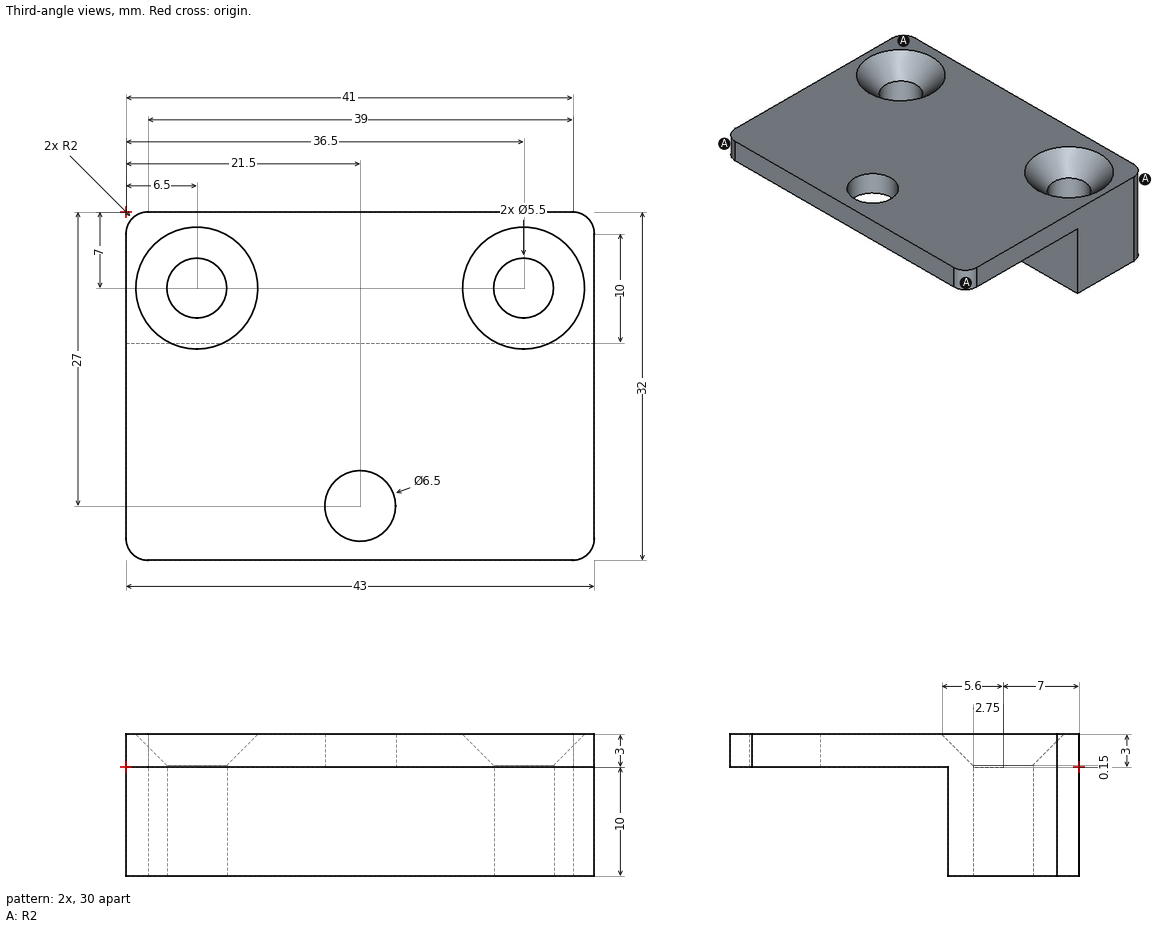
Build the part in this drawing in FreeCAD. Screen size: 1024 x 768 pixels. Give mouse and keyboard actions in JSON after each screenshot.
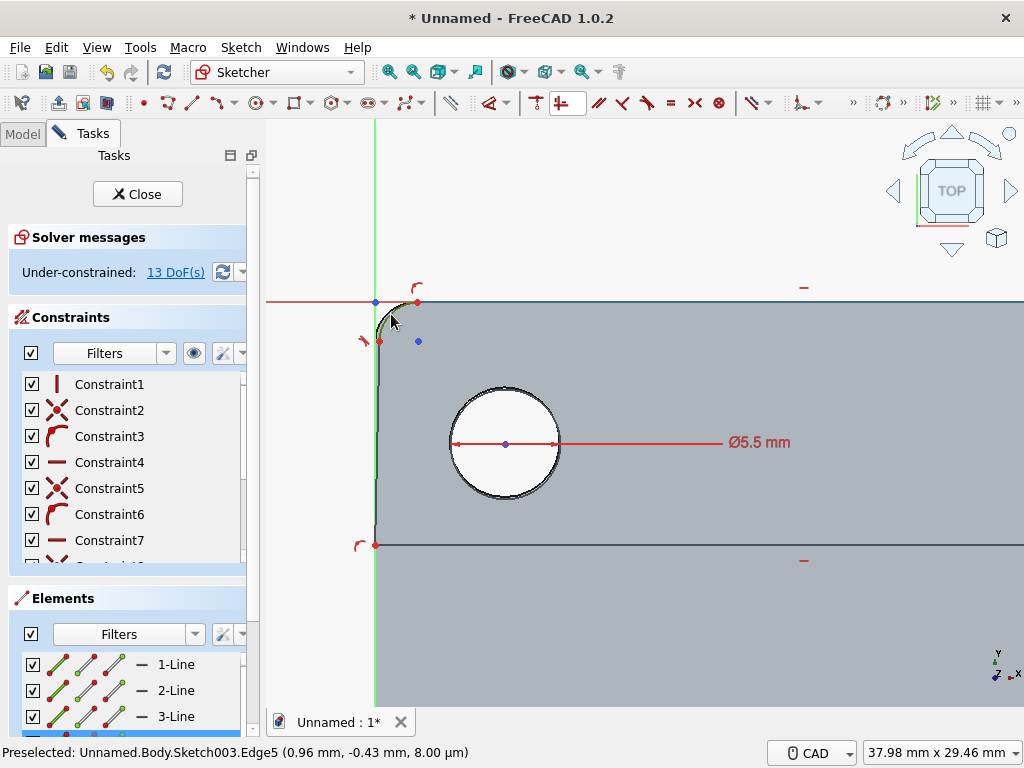
{"action": "left_click", "coordinate": [648, 104]}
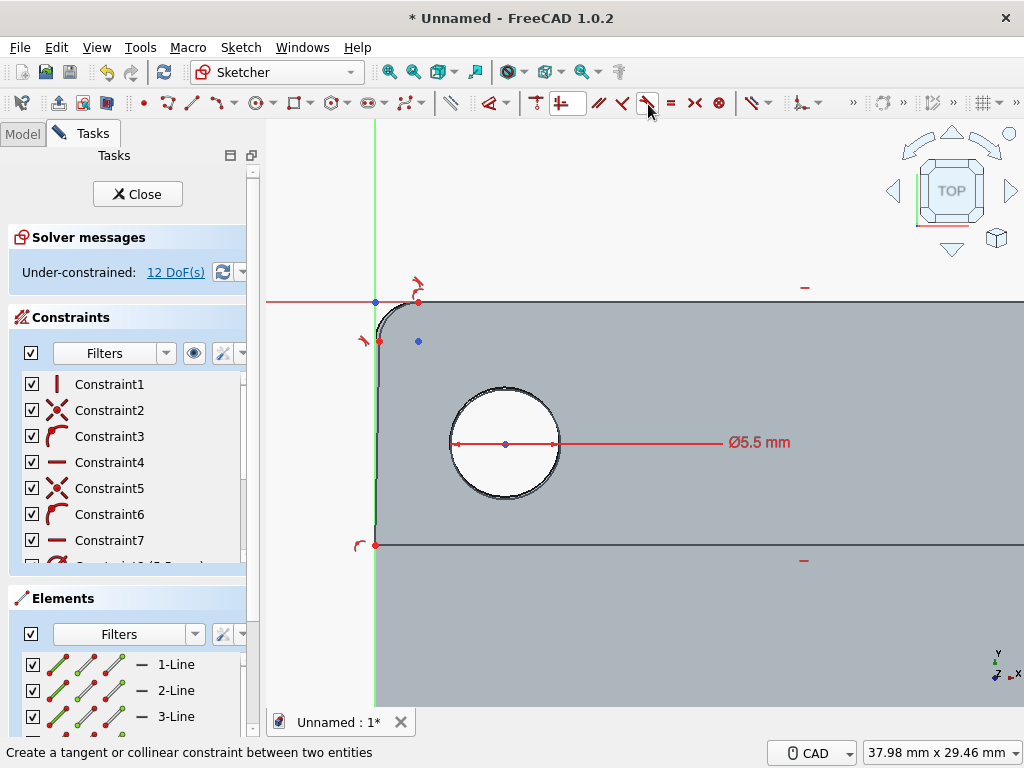
{"action": "left_click", "coordinate": [651, 302]}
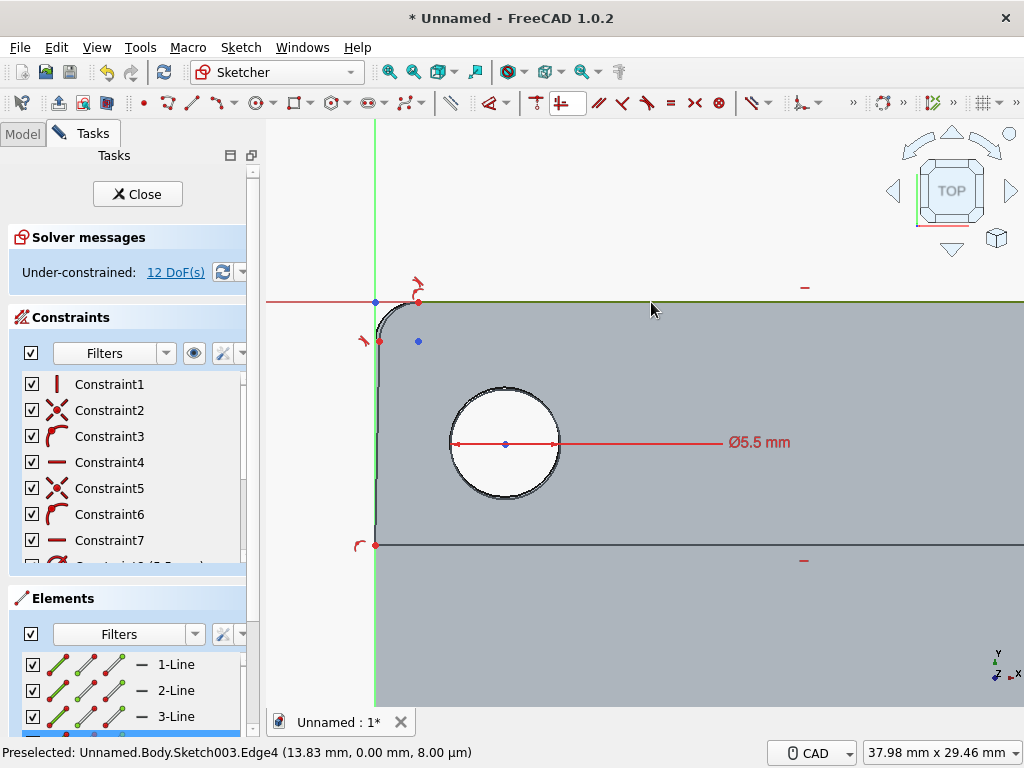
{"action": "scroll", "coordinate": [391, 405], "scroll_direction": "down", "scroll_amount": 4}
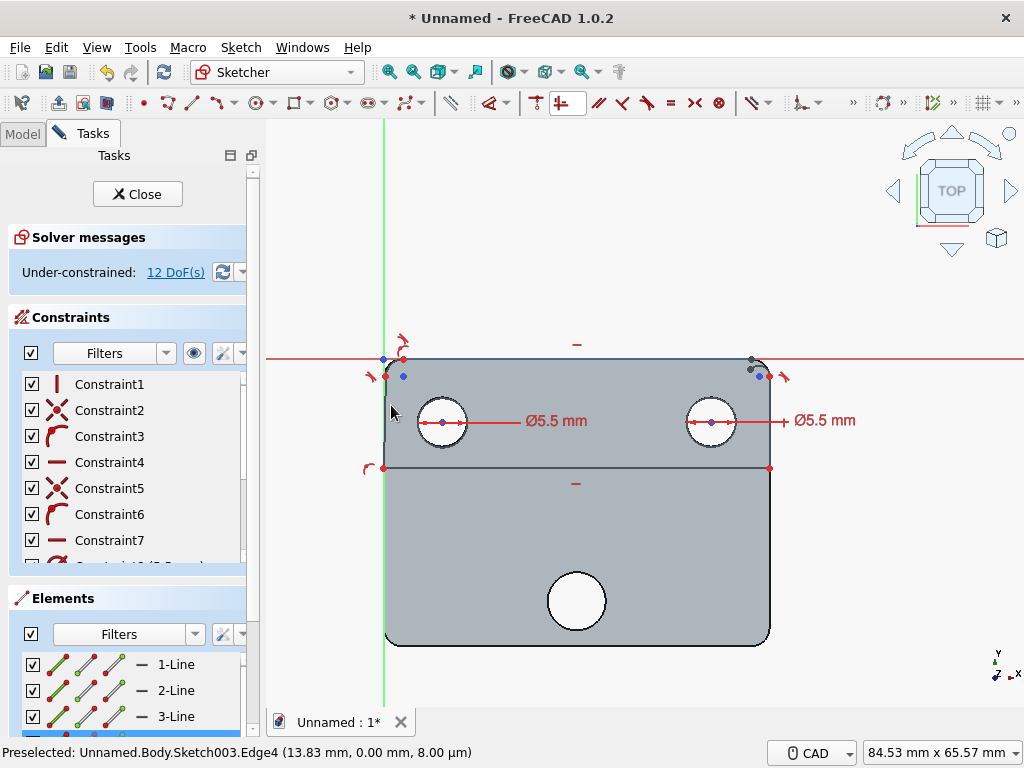
{"action": "scroll", "coordinate": [767, 369], "scroll_direction": "up", "scroll_amount": 3}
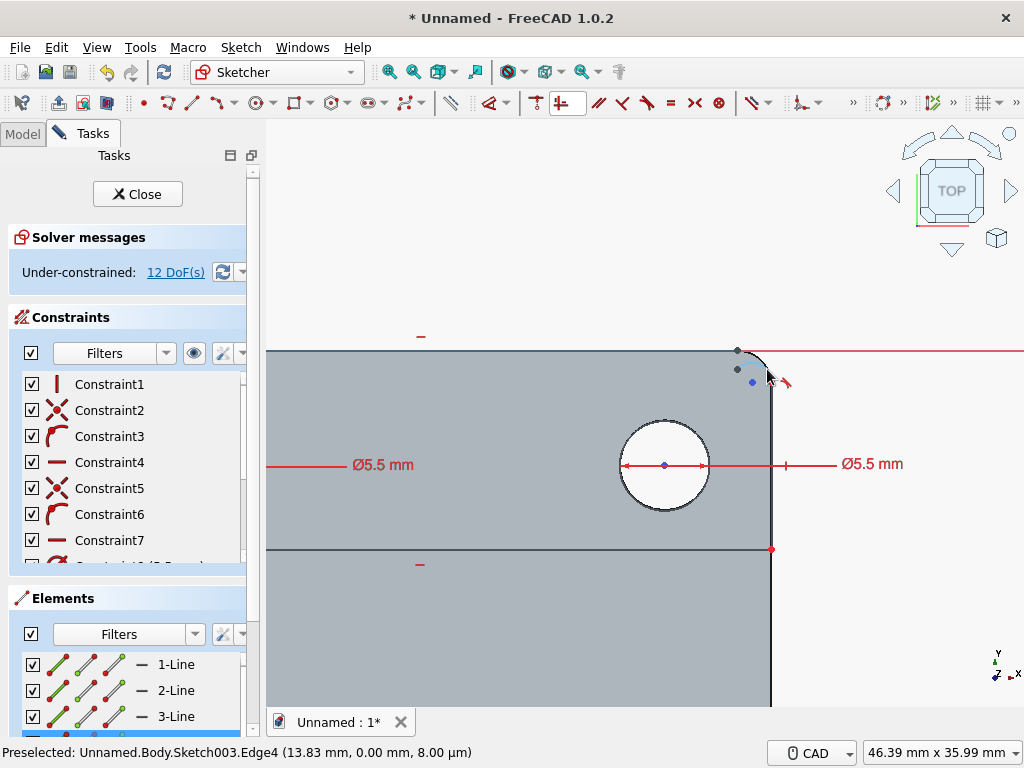
{"action": "left_click", "coordinate": [767, 369]}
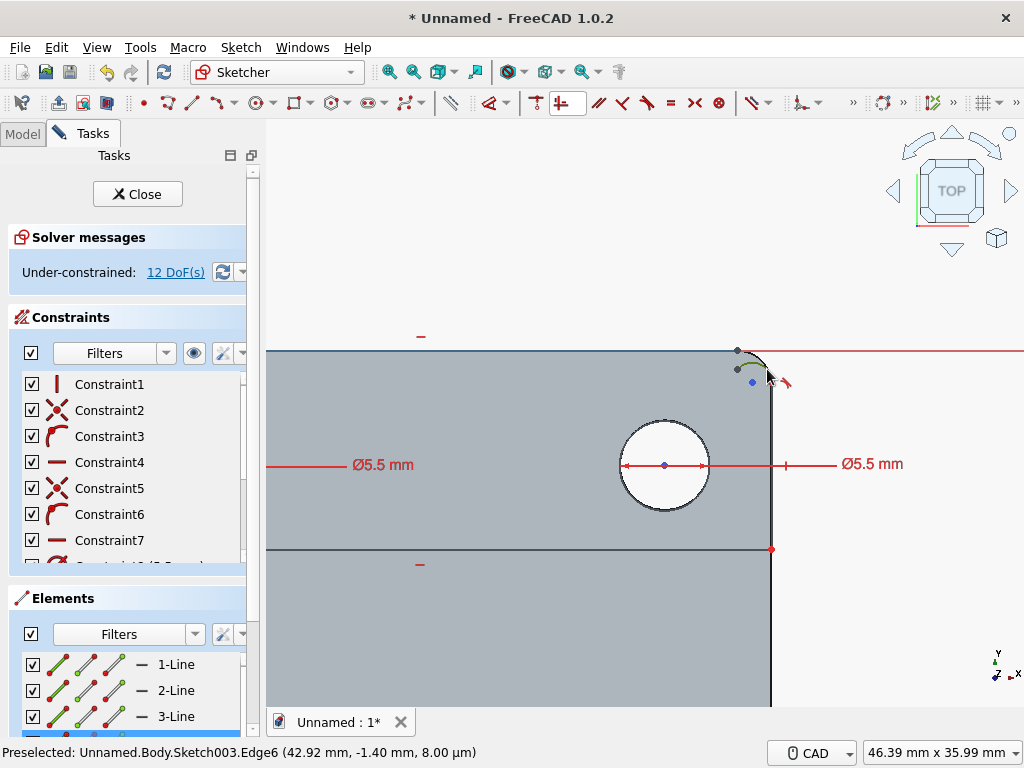
{"action": "left_click", "coordinate": [648, 104]}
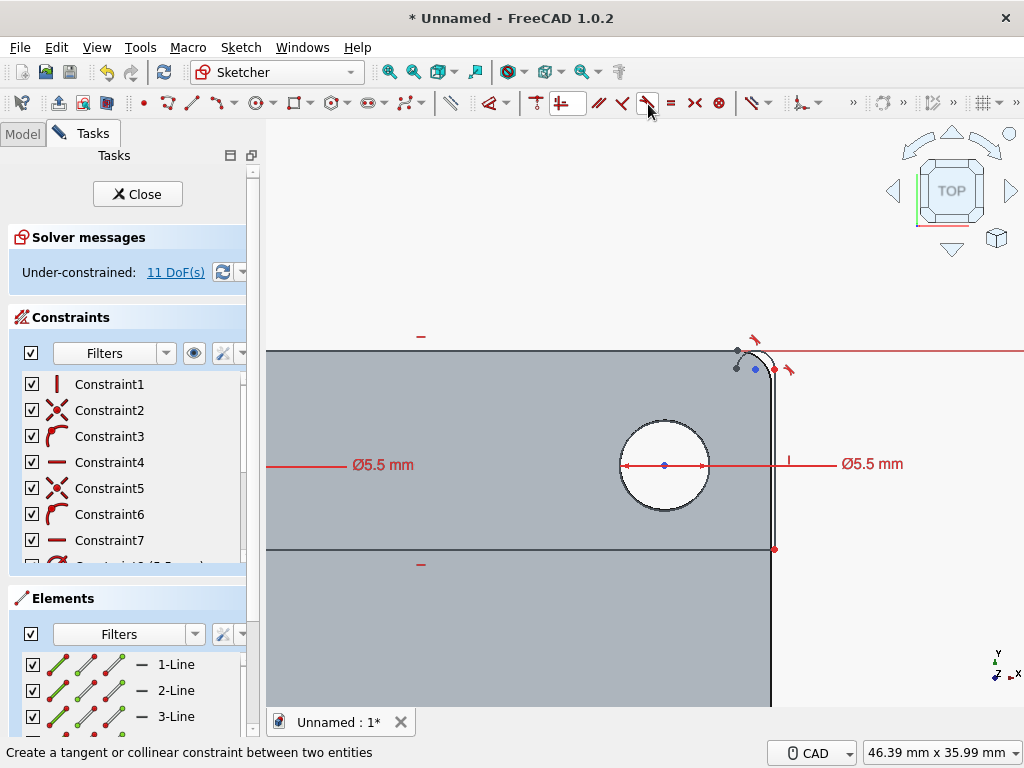
{"action": "scroll", "coordinate": [767, 369], "scroll_direction": "down", "scroll_amount": 3}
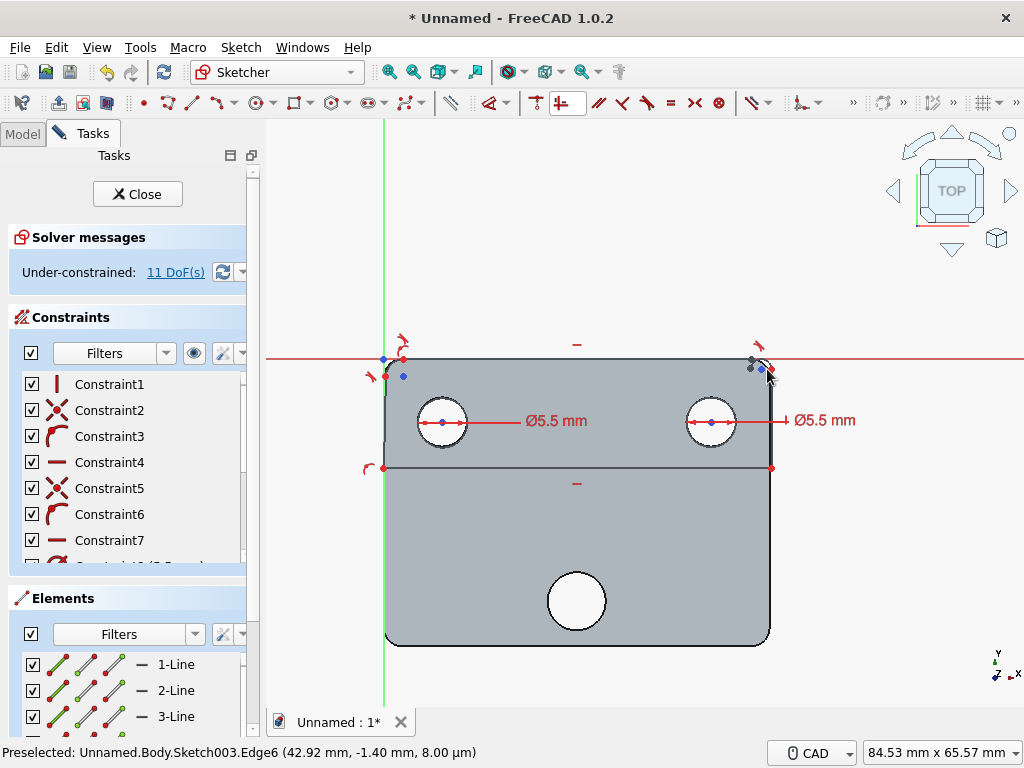
{"action": "left_click", "coordinate": [385, 441]}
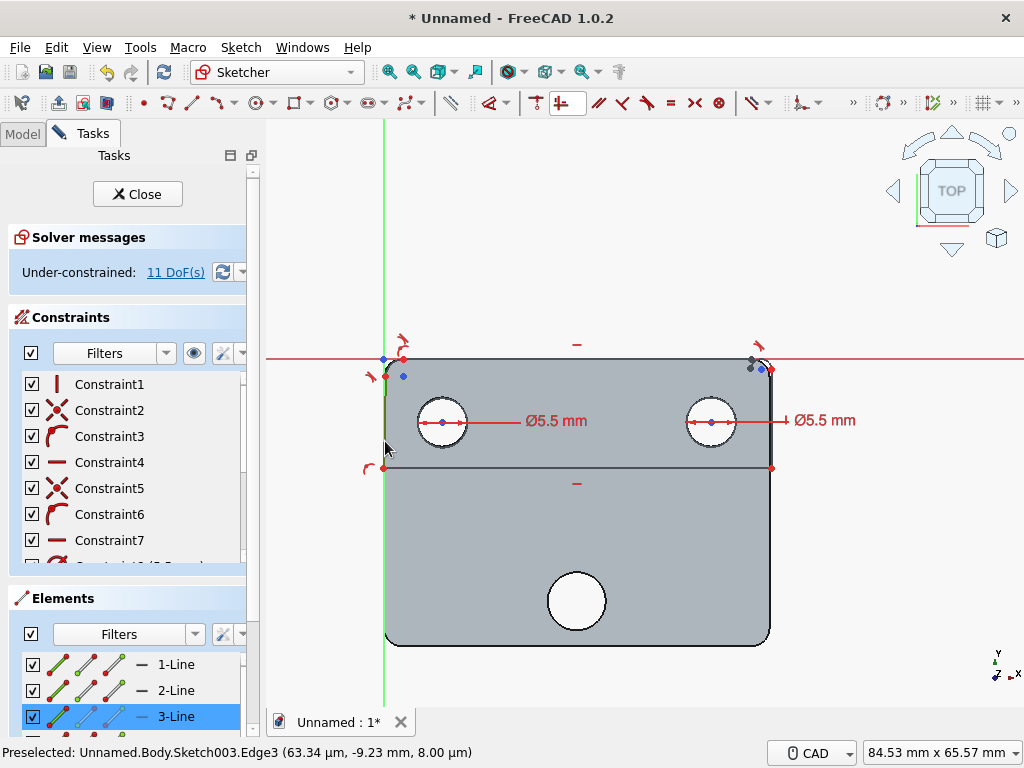
{"action": "left_click", "coordinate": [580, 104]}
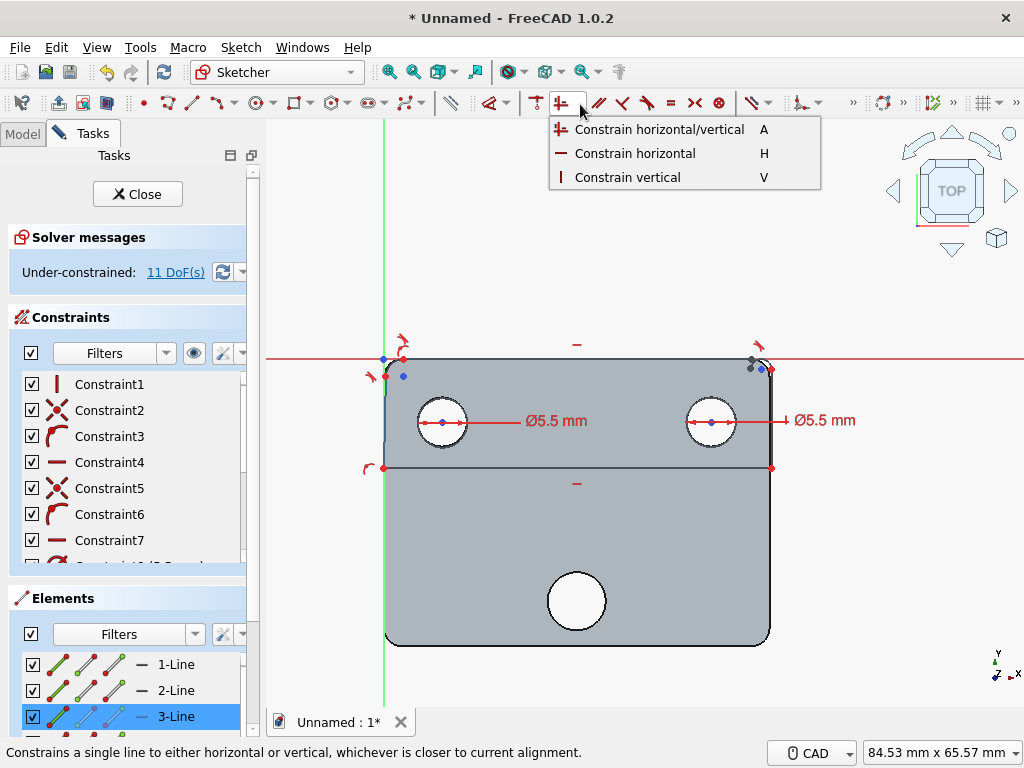
{"action": "left_click", "coordinate": [685, 177]}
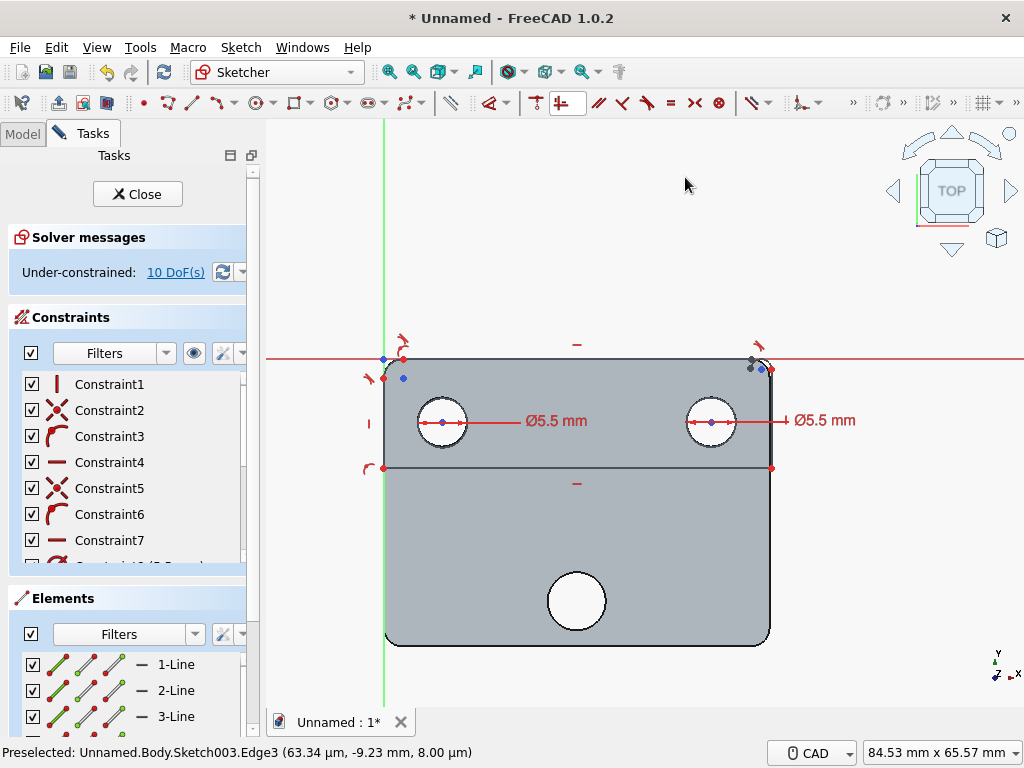
{"action": "scroll", "coordinate": [395, 361], "scroll_direction": "up", "scroll_amount": 3}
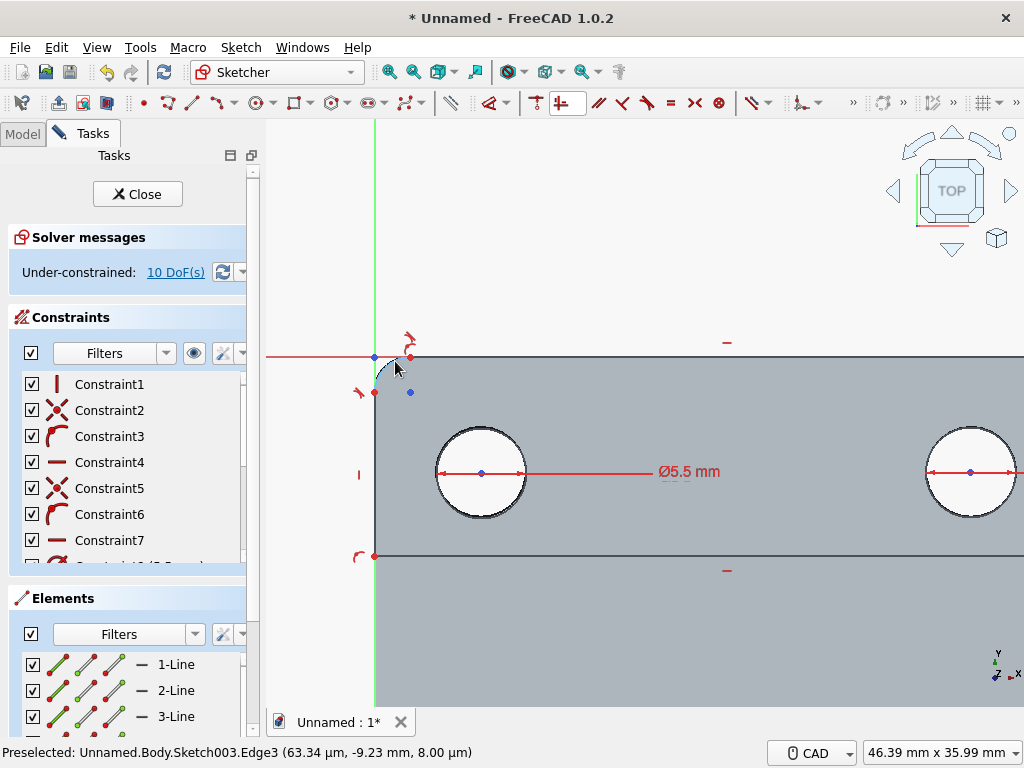
{"action": "left_click", "coordinate": [394, 361]}